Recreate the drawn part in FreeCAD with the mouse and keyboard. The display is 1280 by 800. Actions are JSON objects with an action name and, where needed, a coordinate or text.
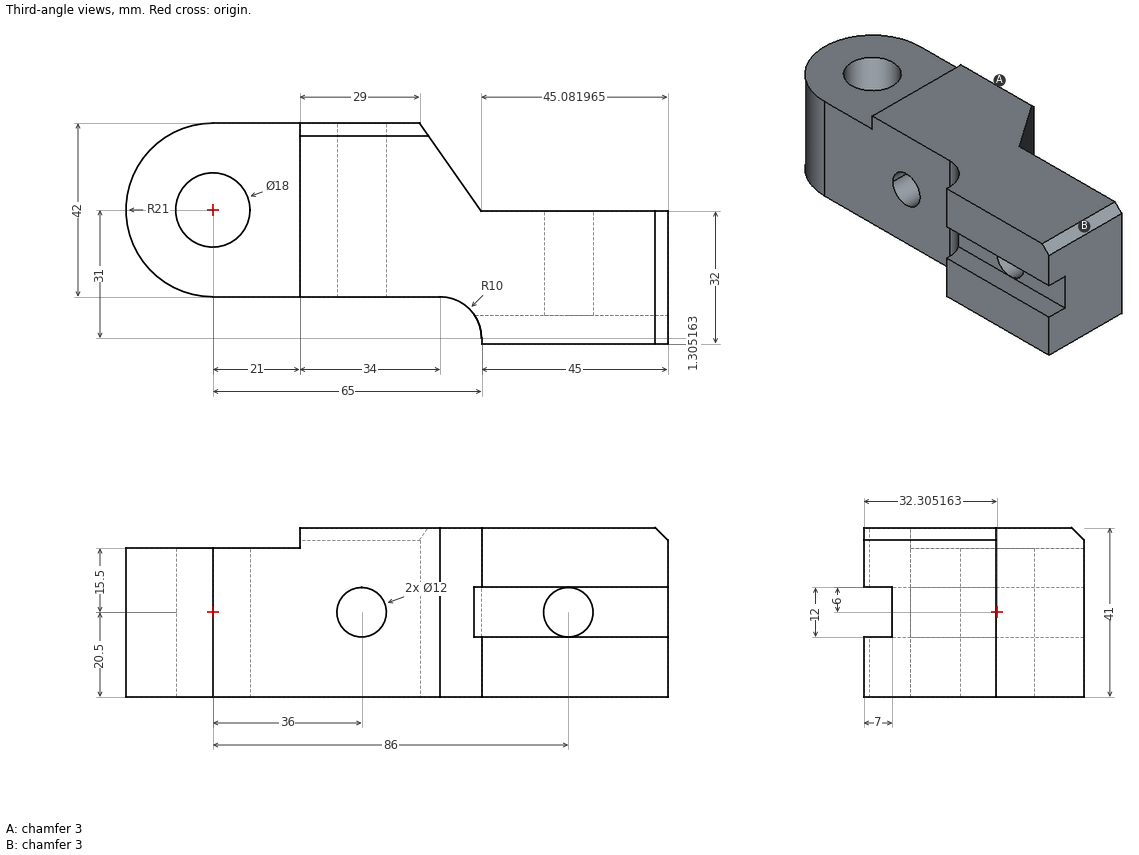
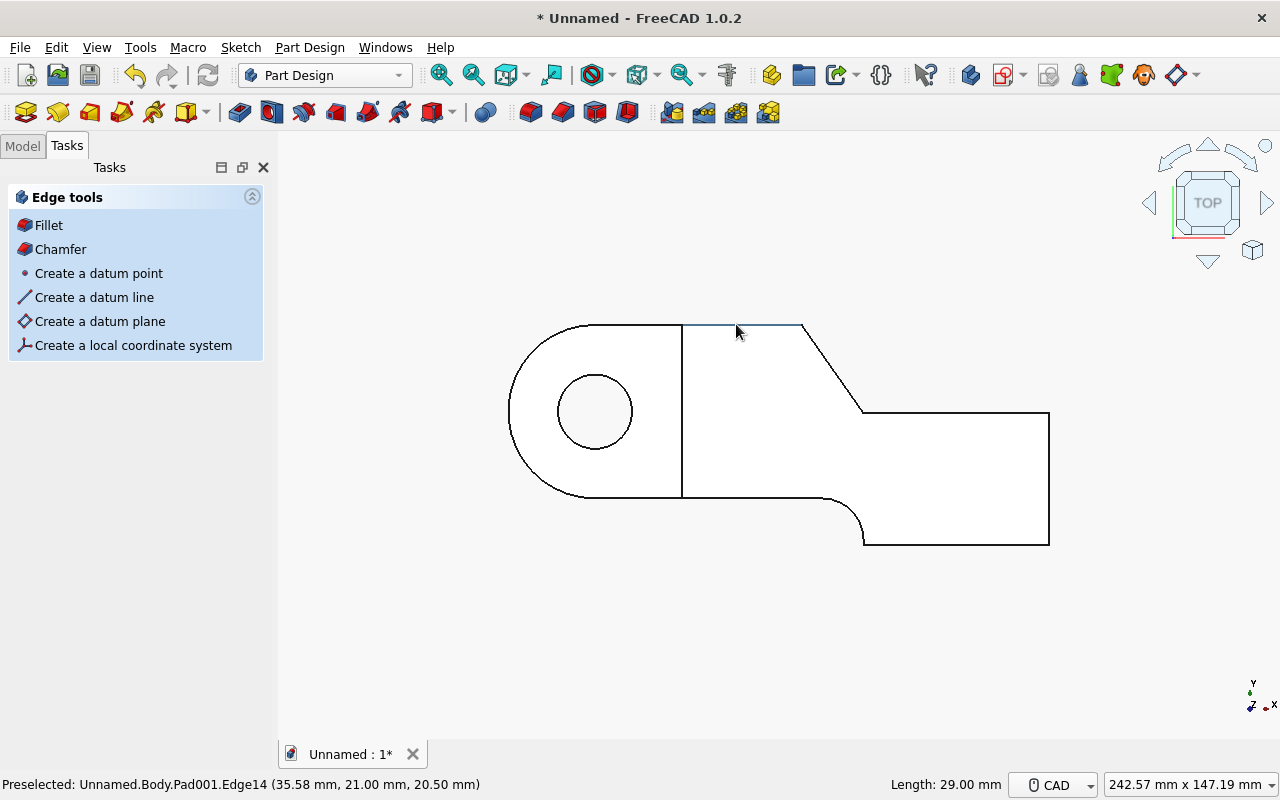
{"action": "left_click", "coordinate": [564, 112]}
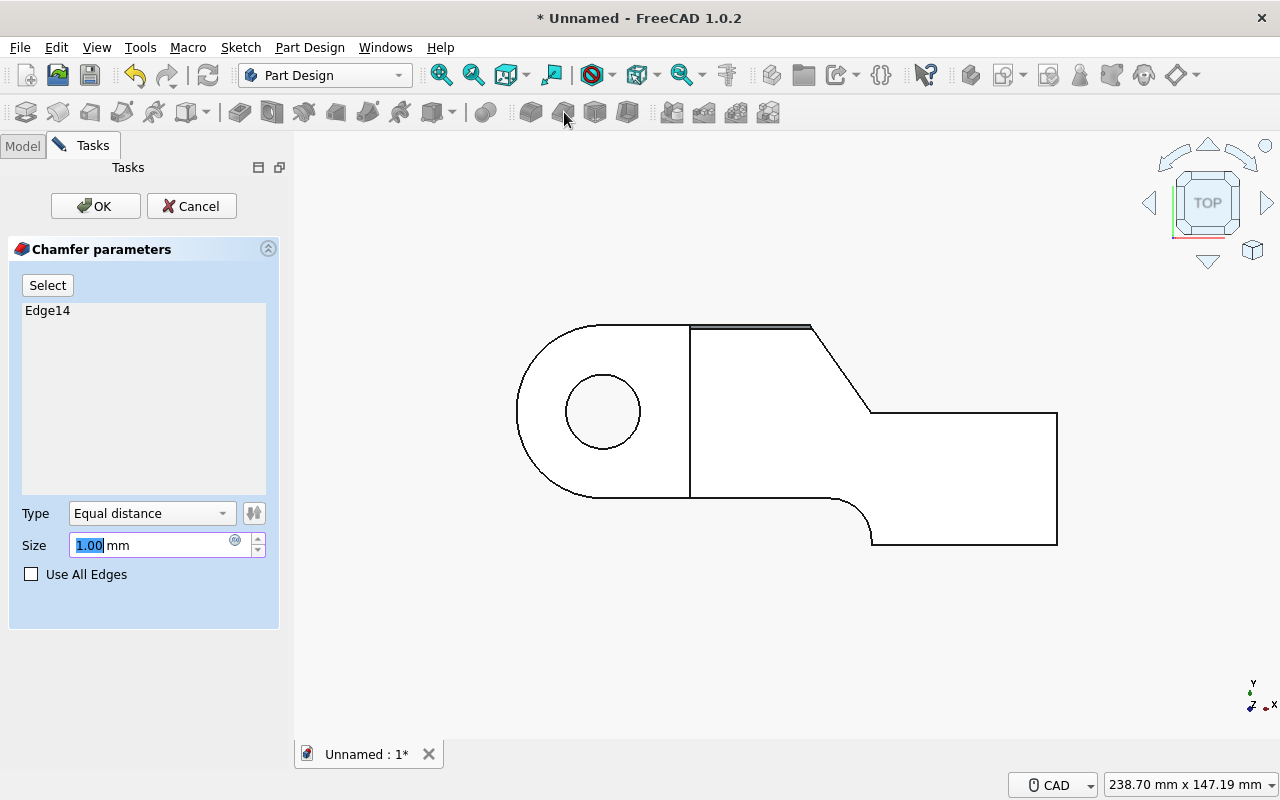
{"action": "type", "text": "3"}
{"action": "key", "text": "Tab"}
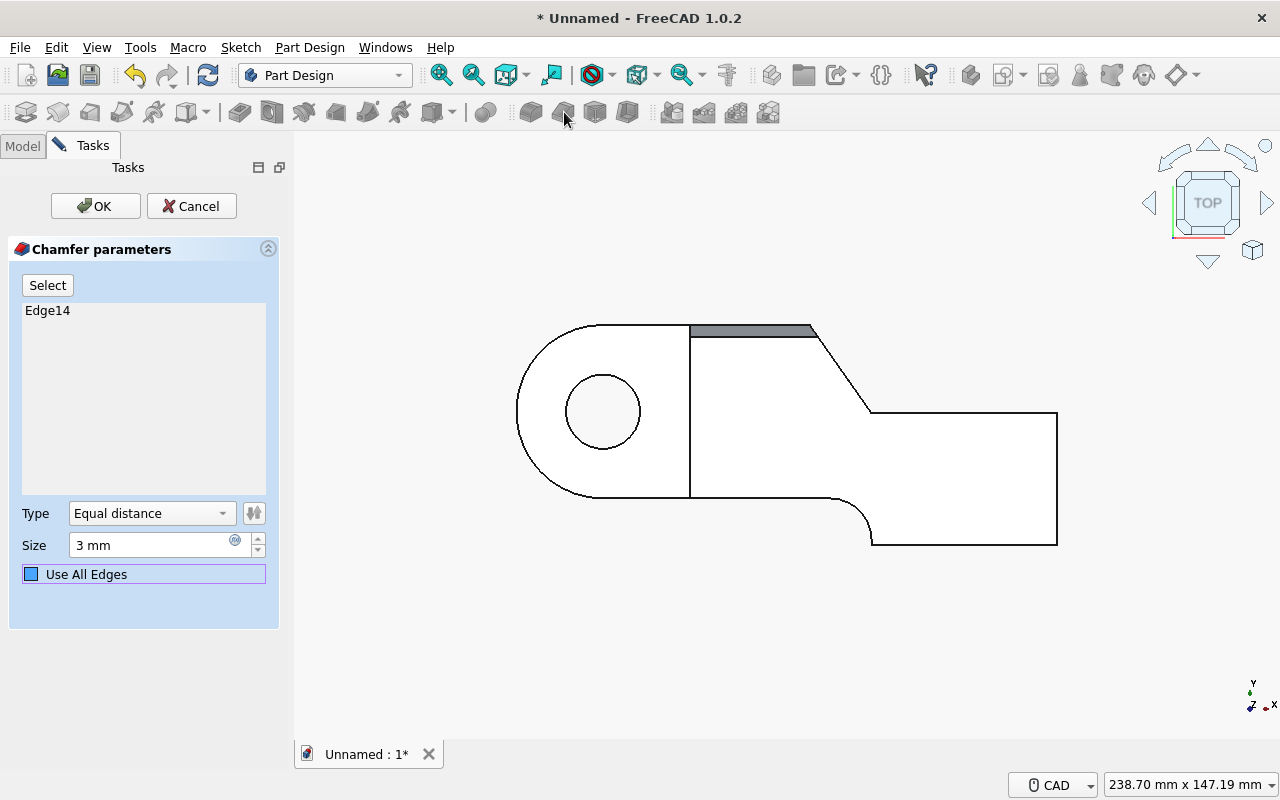
{"action": "left_click", "coordinate": [96, 206]}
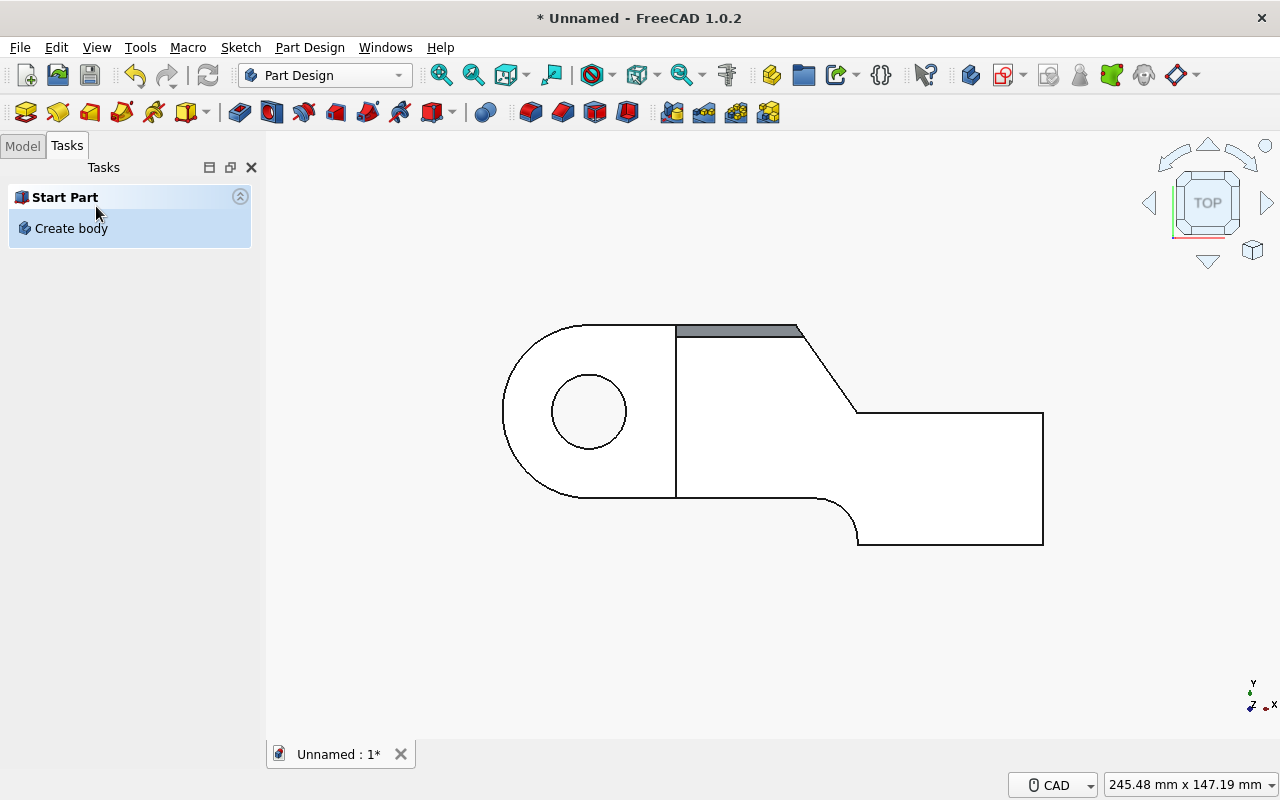
{"action": "left_click", "coordinate": [1043, 478]}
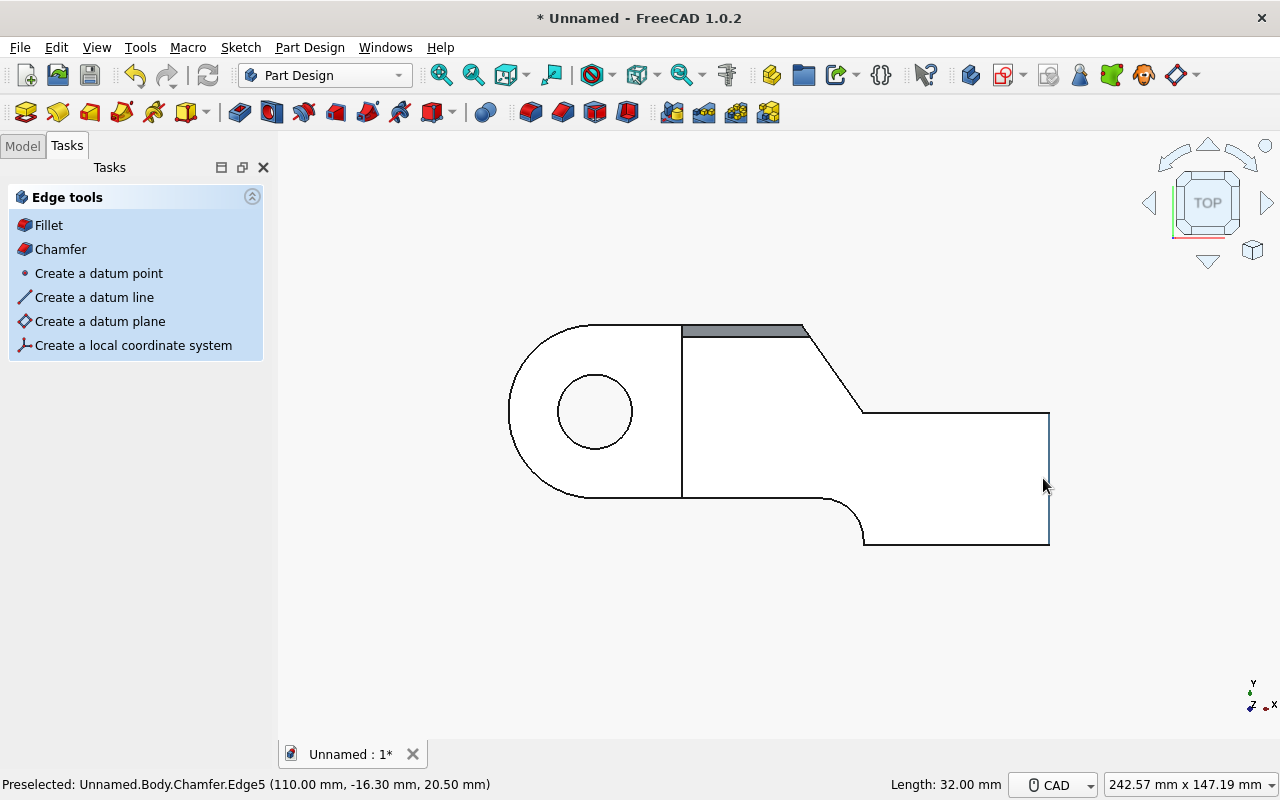
{"action": "left_click", "coordinate": [564, 112]}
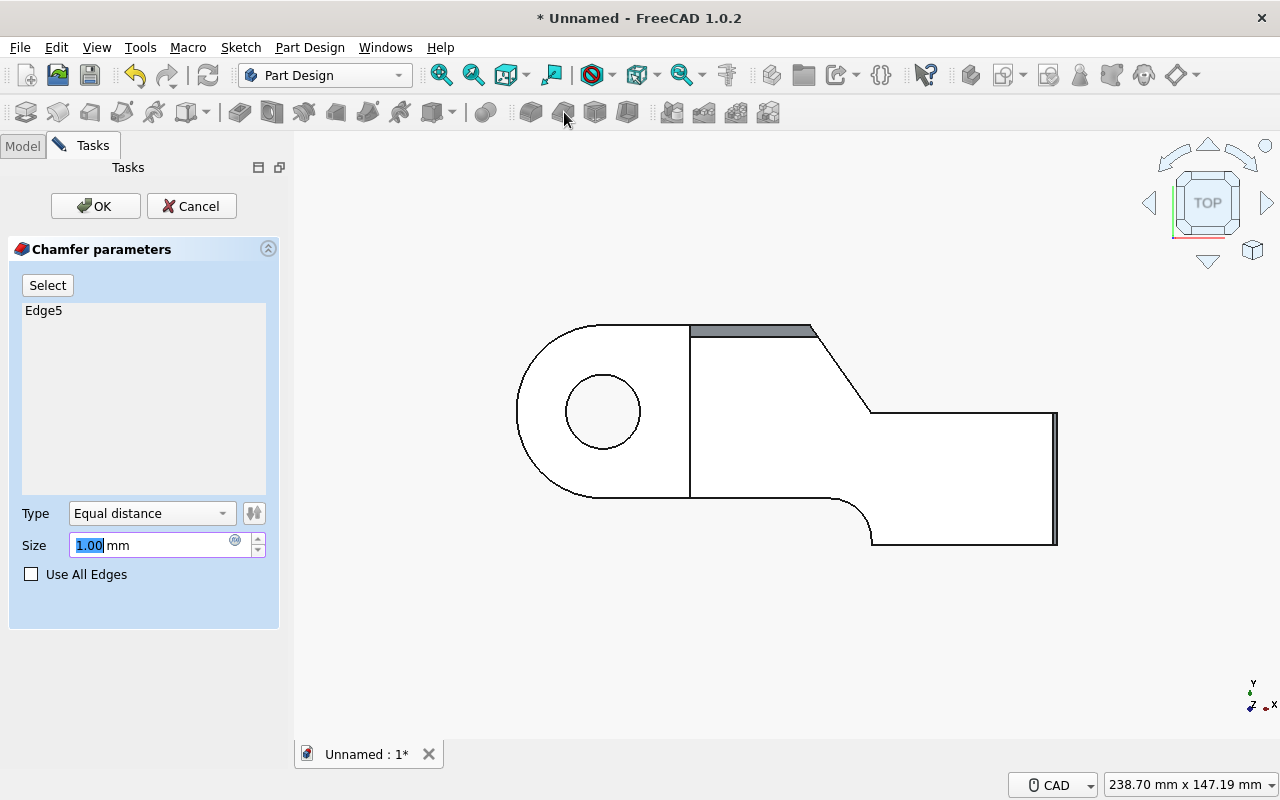
{"action": "type", "text": "3"}
{"action": "key", "text": "Tab"}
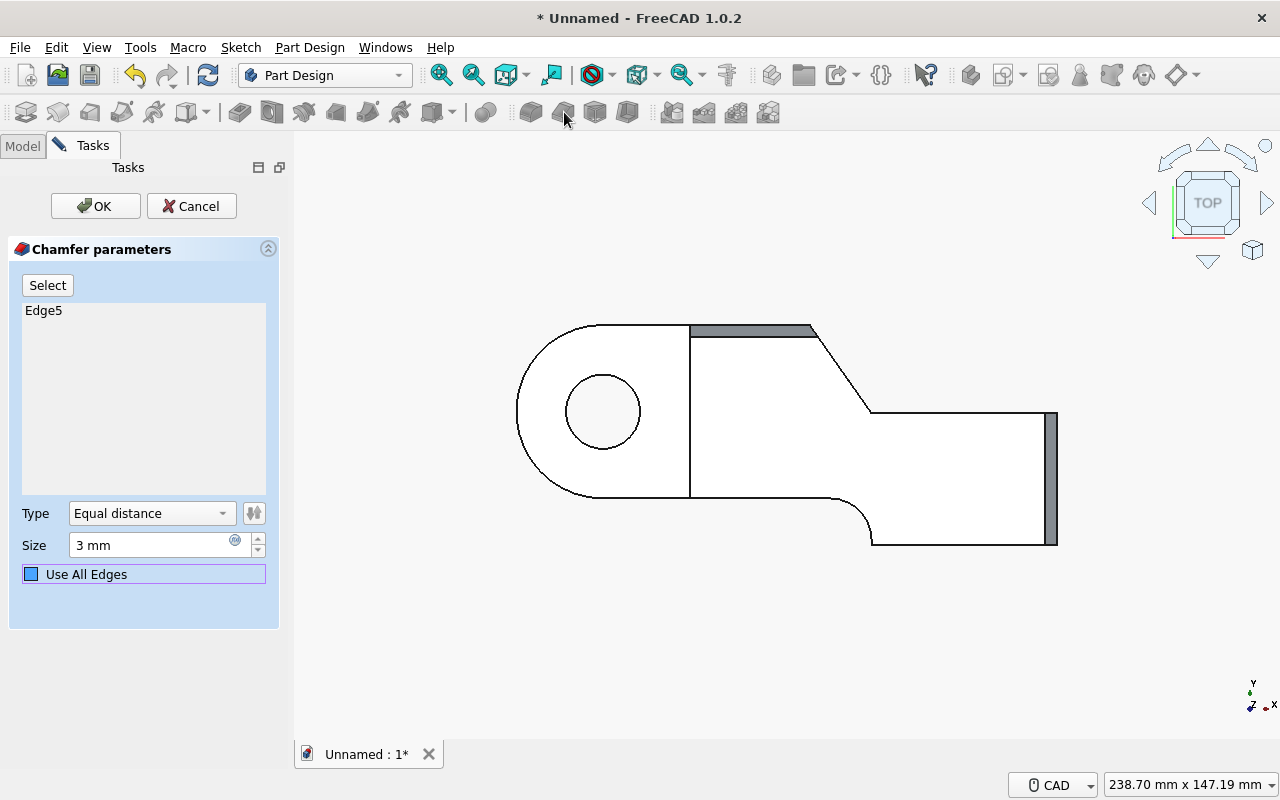
{"action": "left_click", "coordinate": [96, 206]}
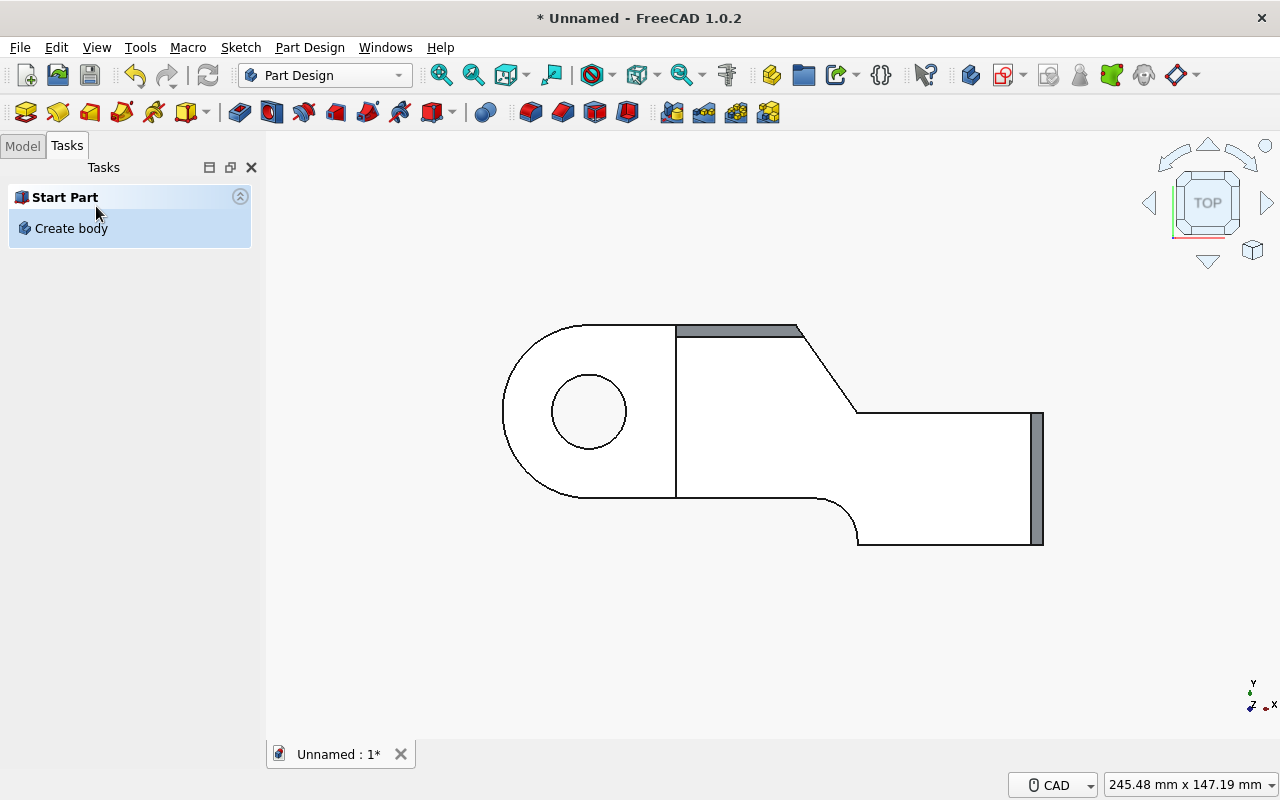
{"action": "key", "text": "0"}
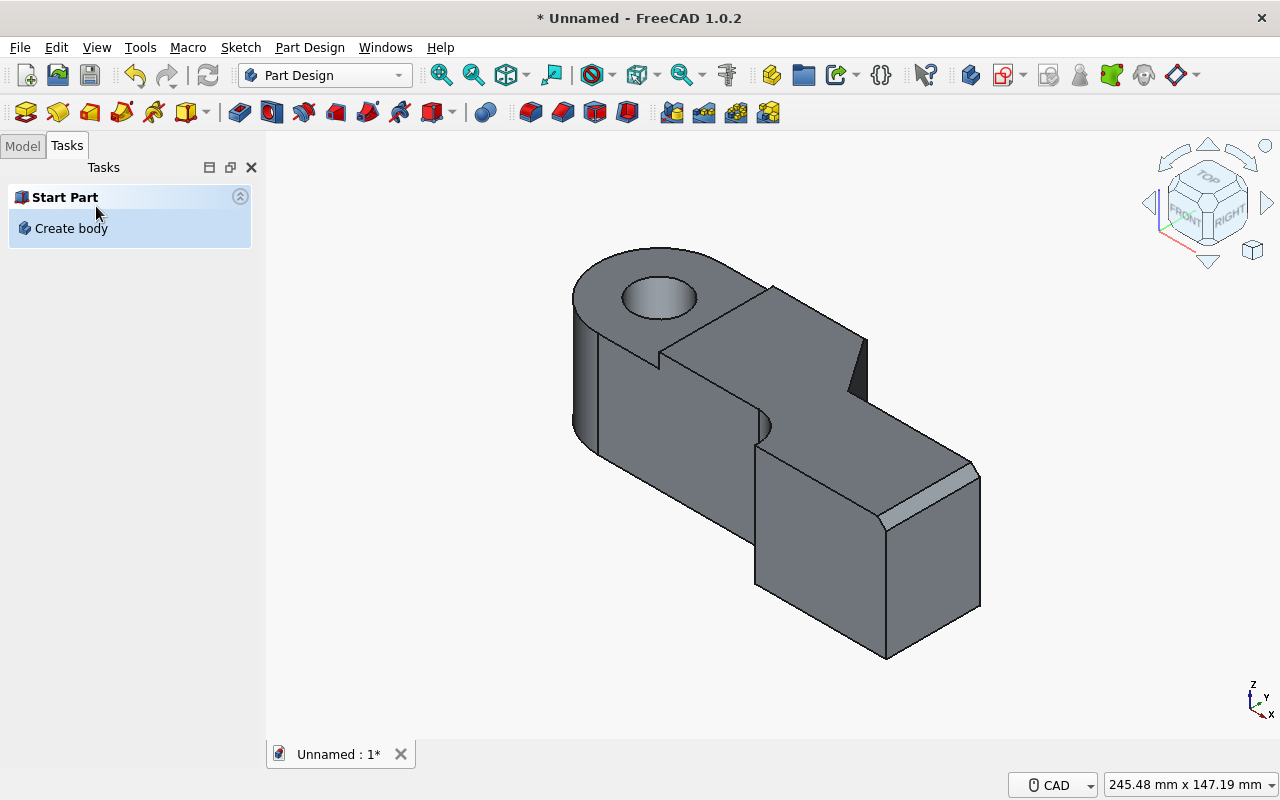
{"action": "left_click", "coordinate": [933, 567]}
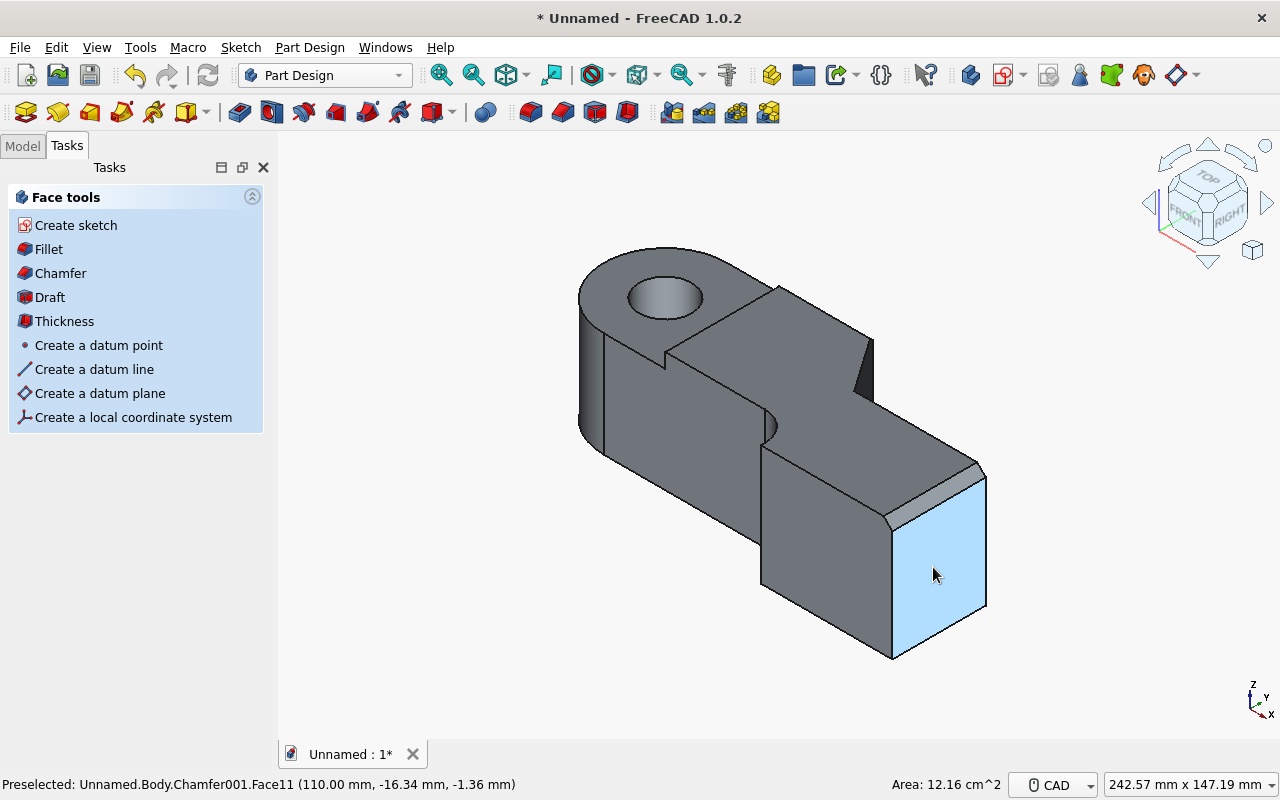
{"action": "left_click", "coordinate": [1004, 76]}